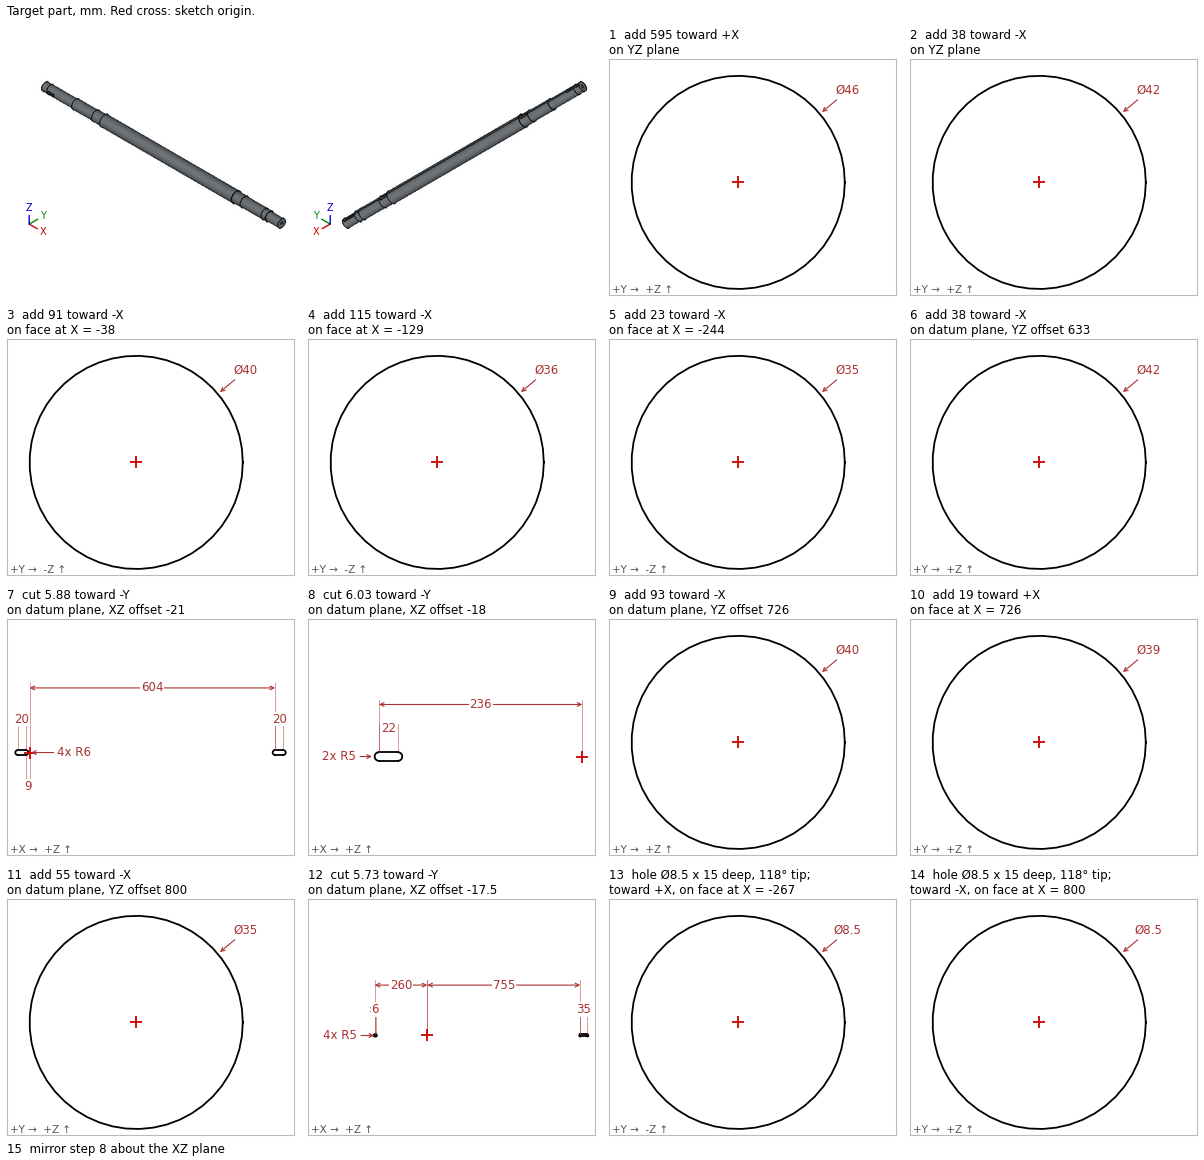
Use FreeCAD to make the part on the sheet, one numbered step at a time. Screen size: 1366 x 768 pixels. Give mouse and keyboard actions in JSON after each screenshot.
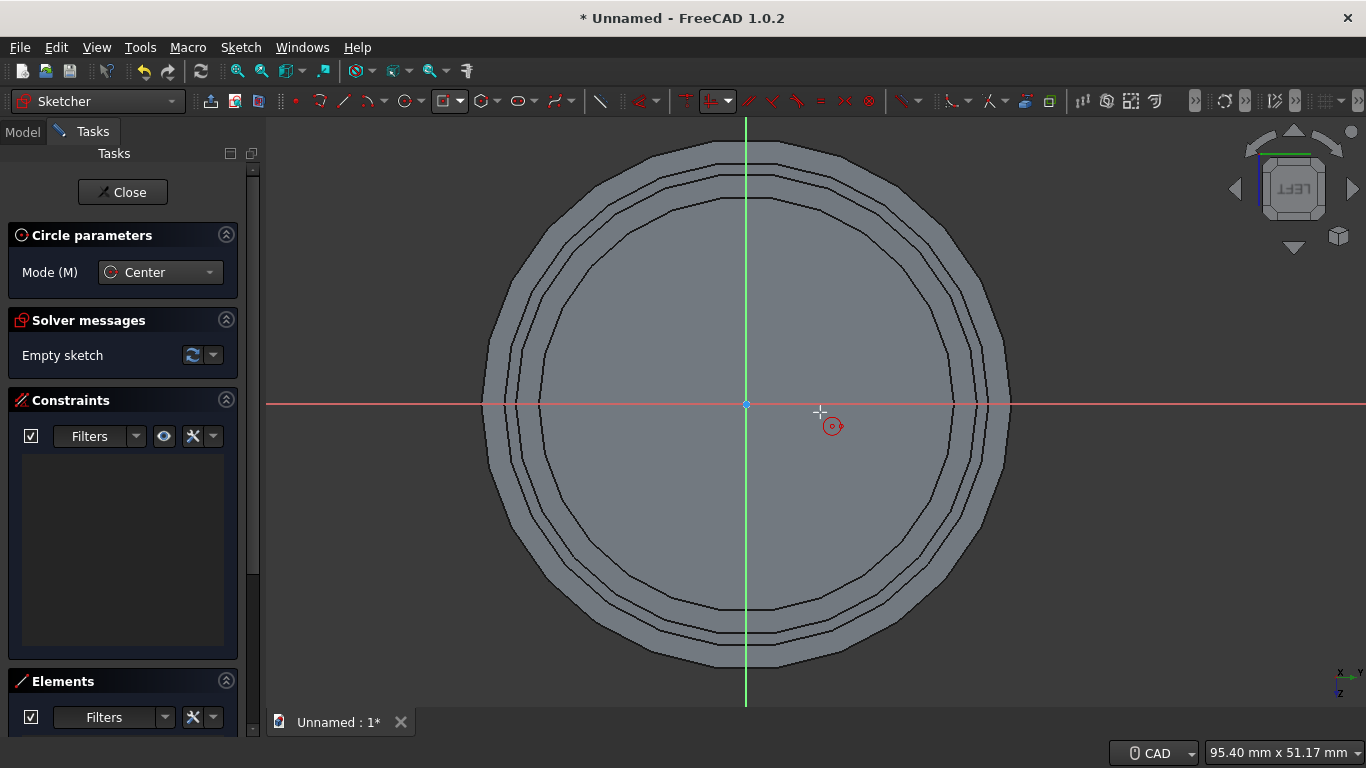
{"action": "left_click", "coordinate": [746, 404]}
{"action": "mouse_move", "coordinate": [889, 262]}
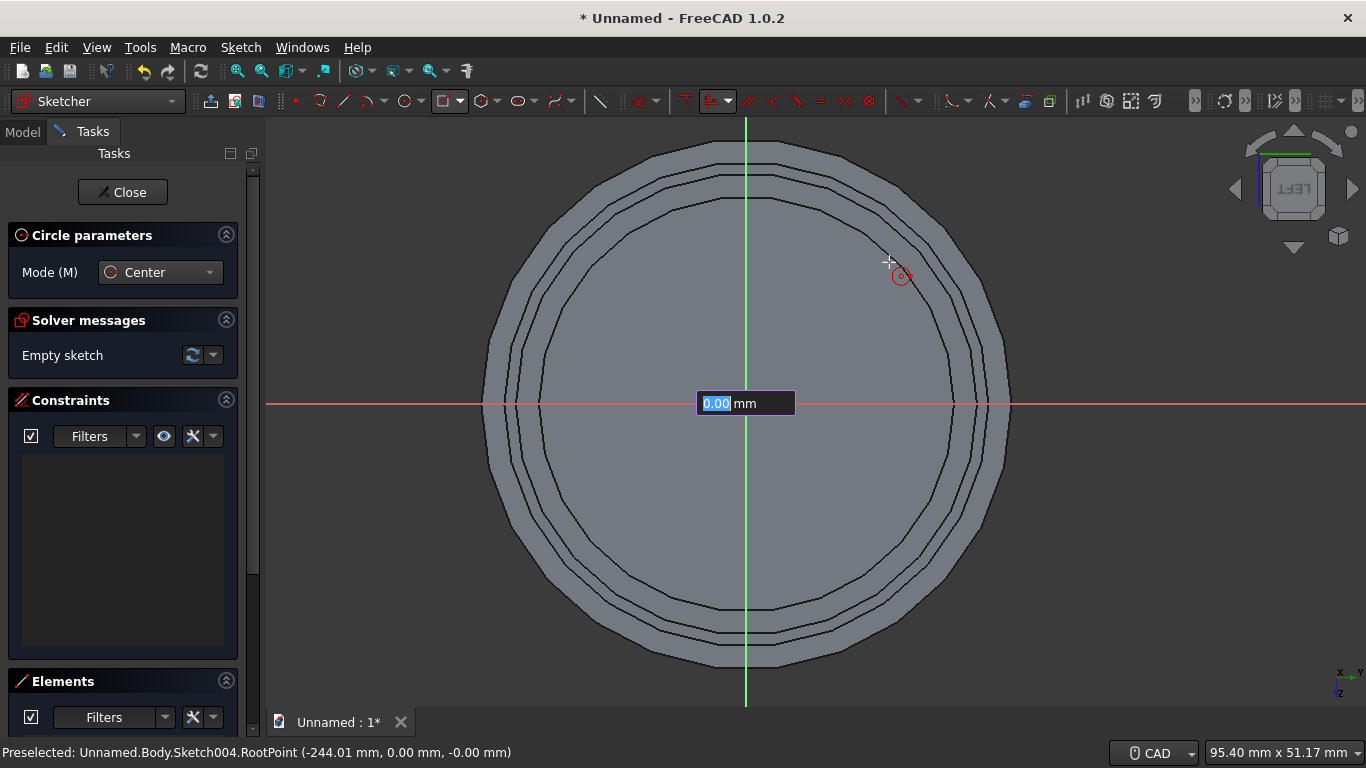
{"action": "type", "text": "35"}
{"action": "key", "text": "Return"}
{"action": "key", "text": "Escape"}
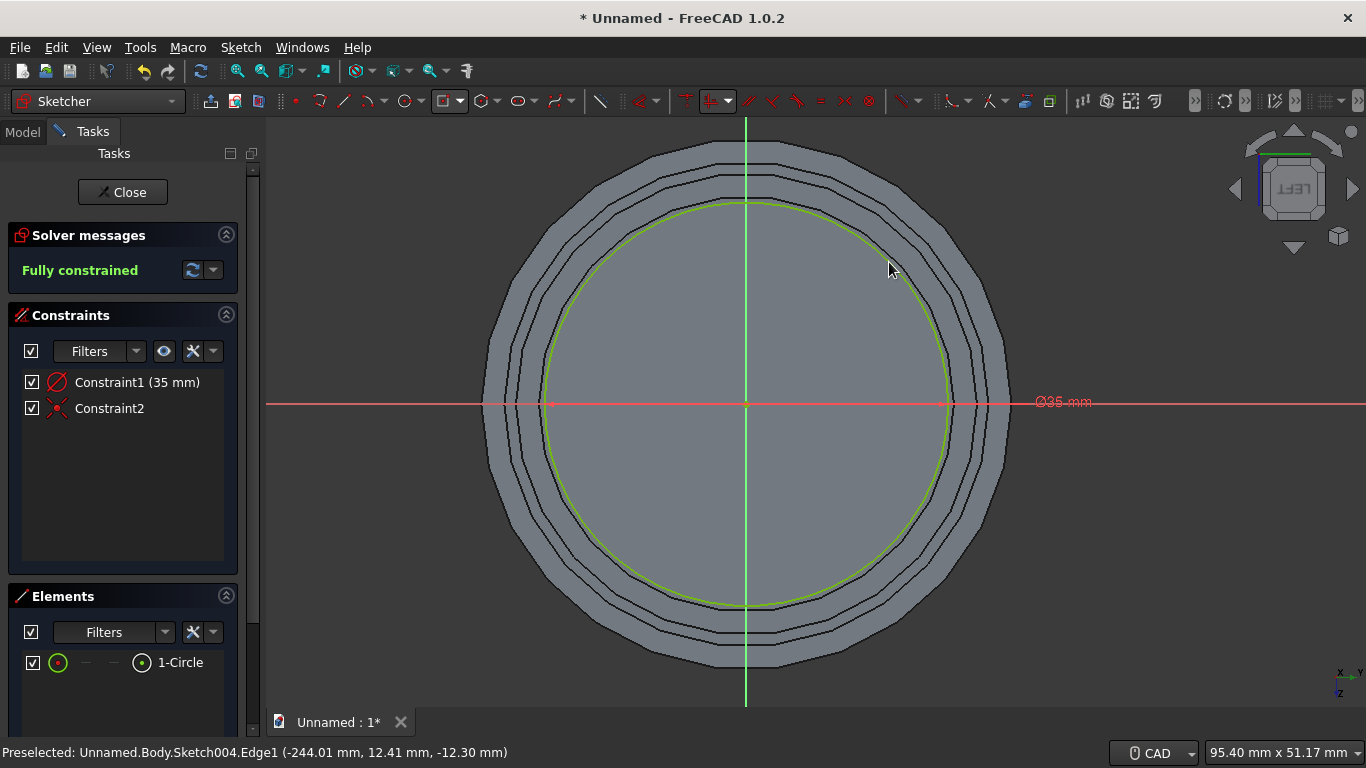
{"action": "left_click", "coordinate": [123, 192]}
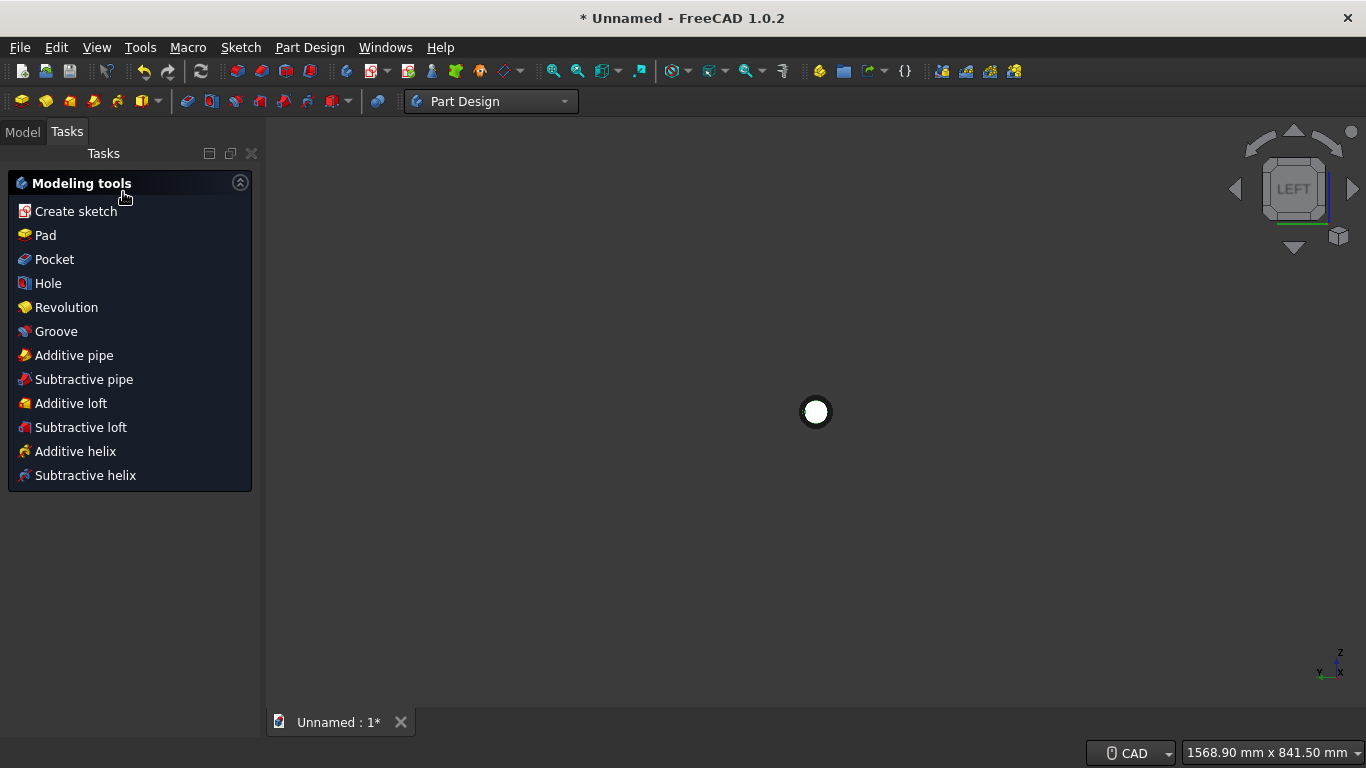
{"action": "left_click", "coordinate": [22, 102]}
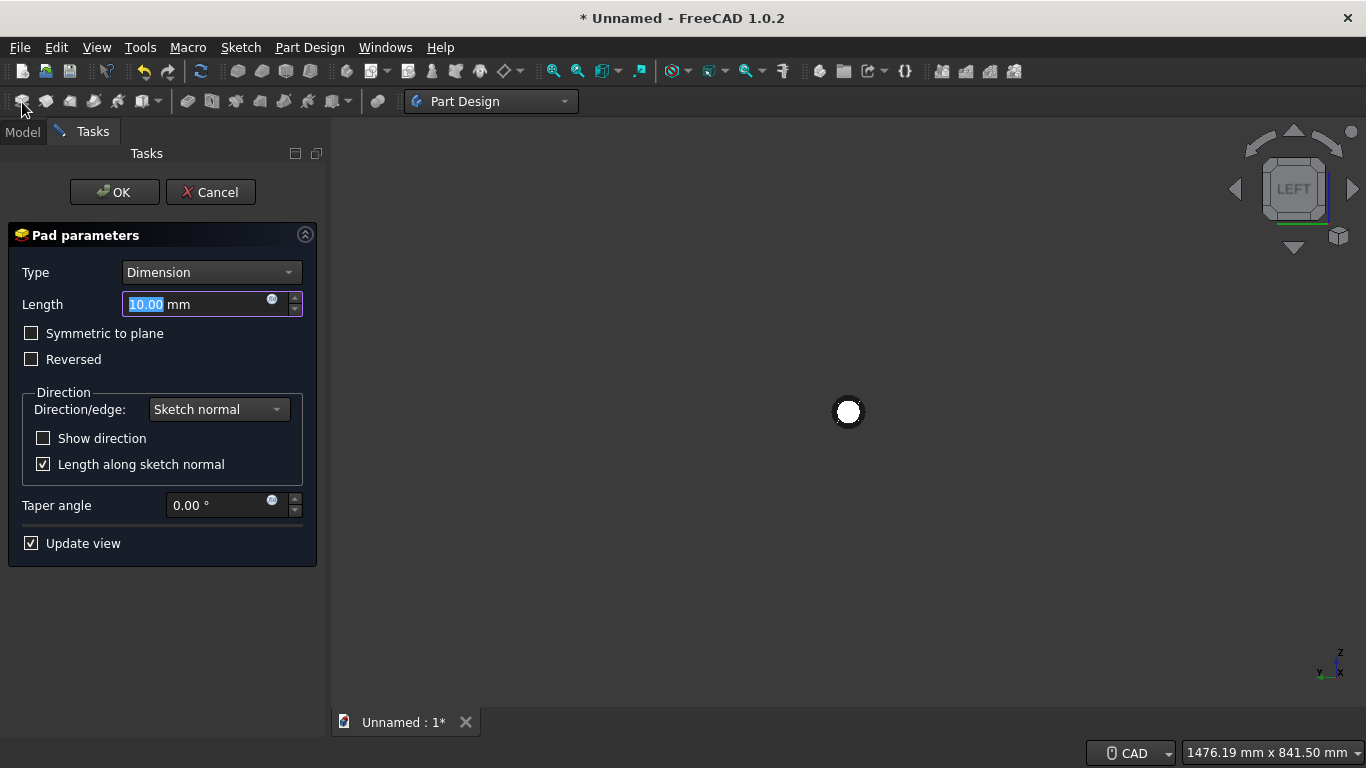
{"action": "type", "text": "23"}
{"action": "key", "text": "Tab"}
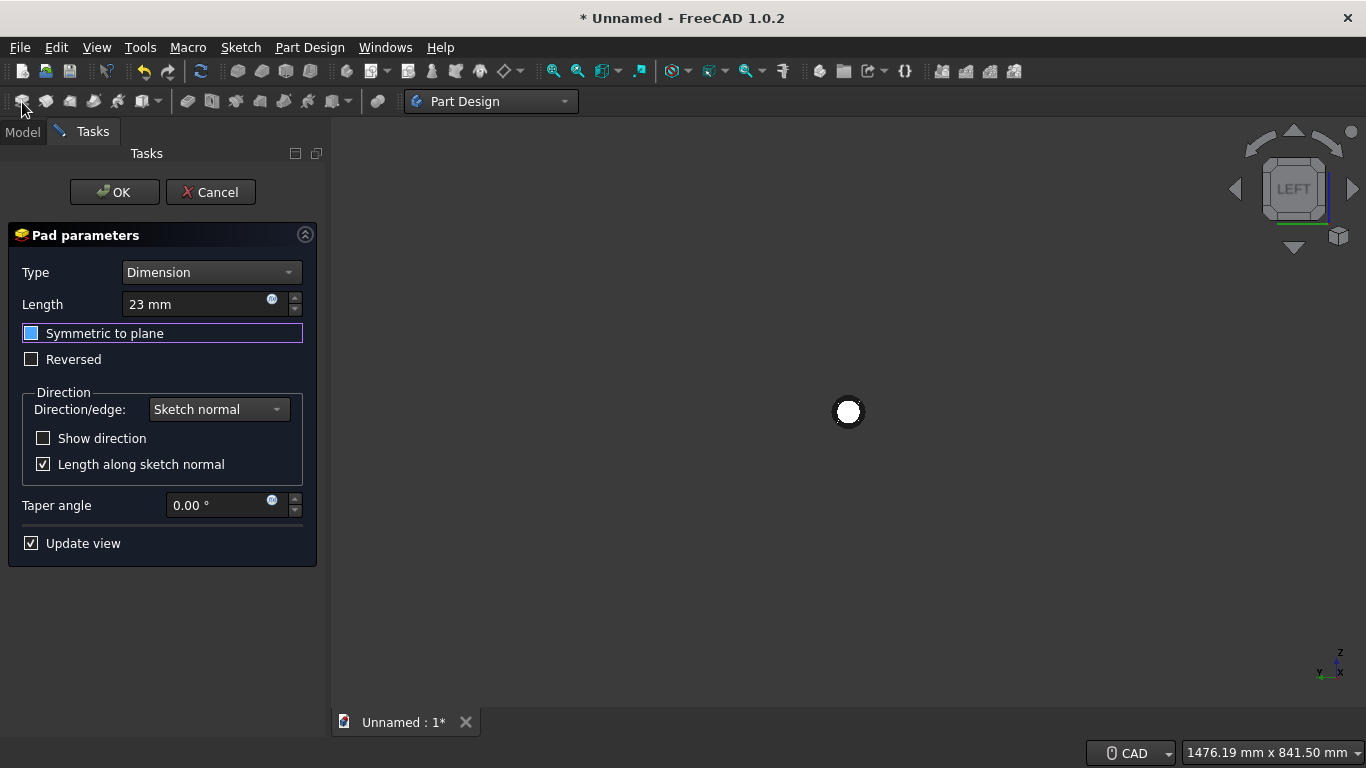
{"action": "left_click", "coordinate": [115, 192]}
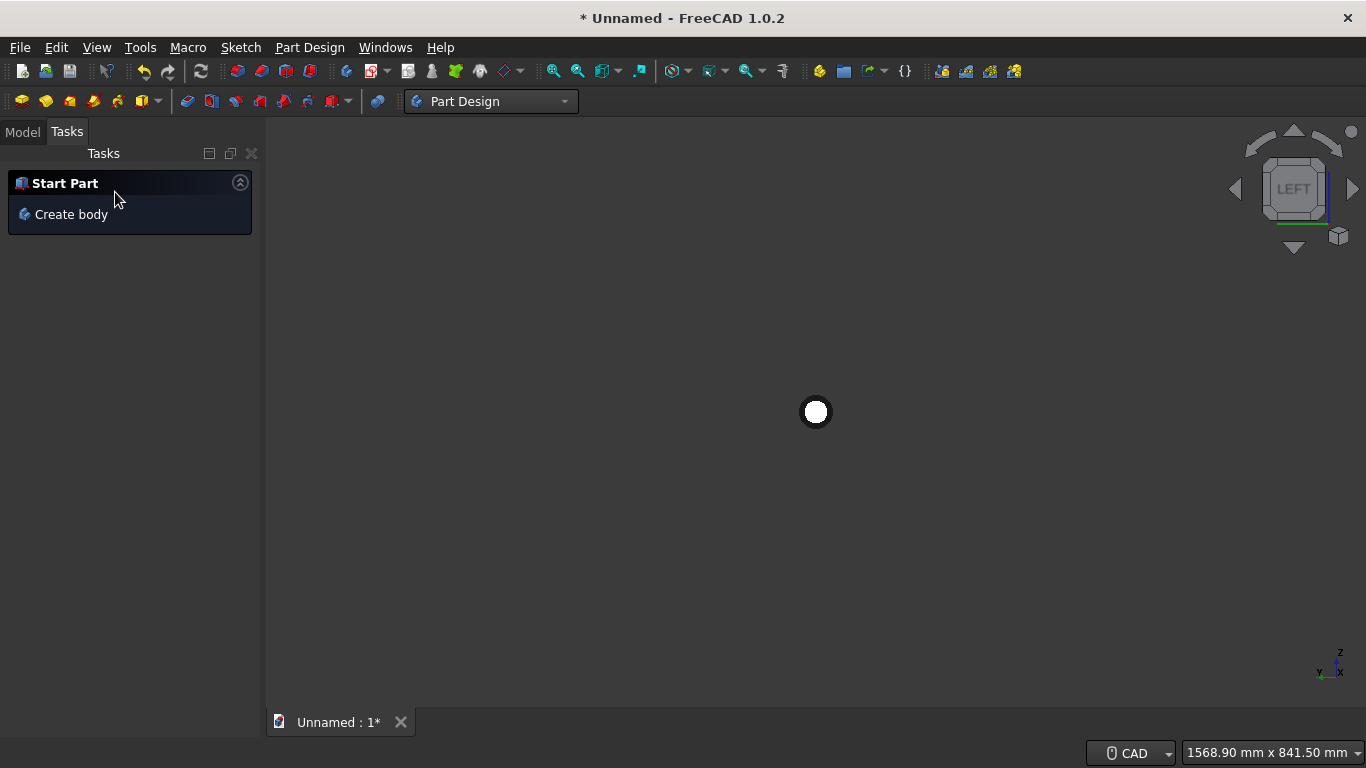
{"action": "key", "text": "v f"}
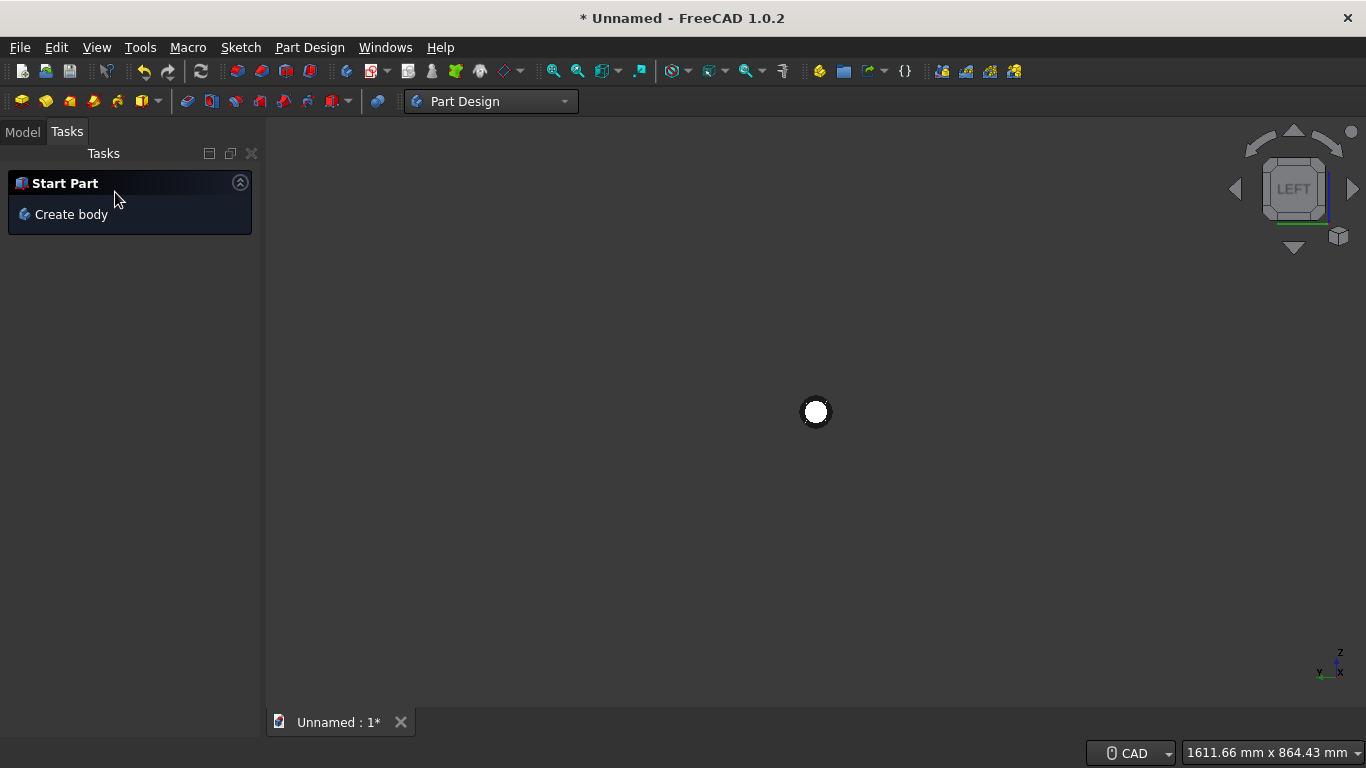
{"action": "left_click", "coordinate": [23, 131]}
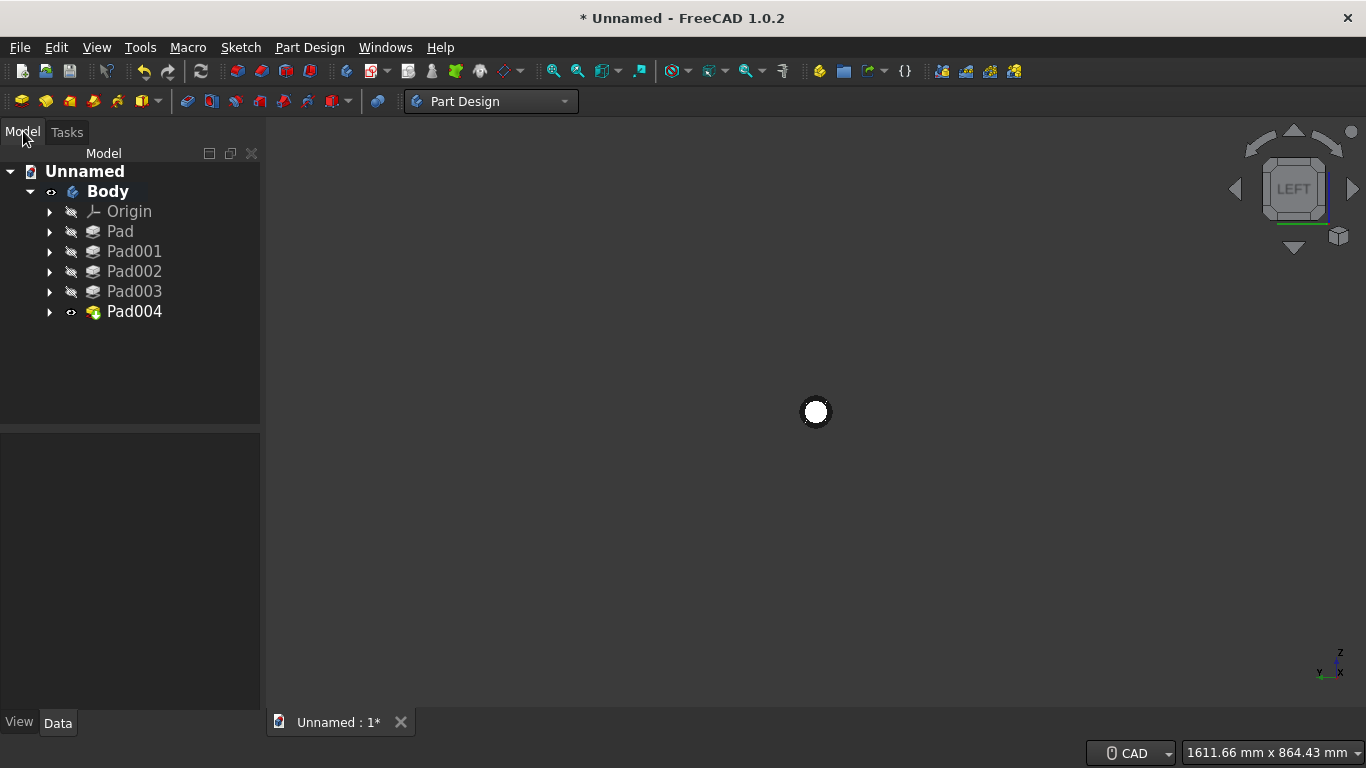
{"action": "left_click", "coordinate": [50, 212]}